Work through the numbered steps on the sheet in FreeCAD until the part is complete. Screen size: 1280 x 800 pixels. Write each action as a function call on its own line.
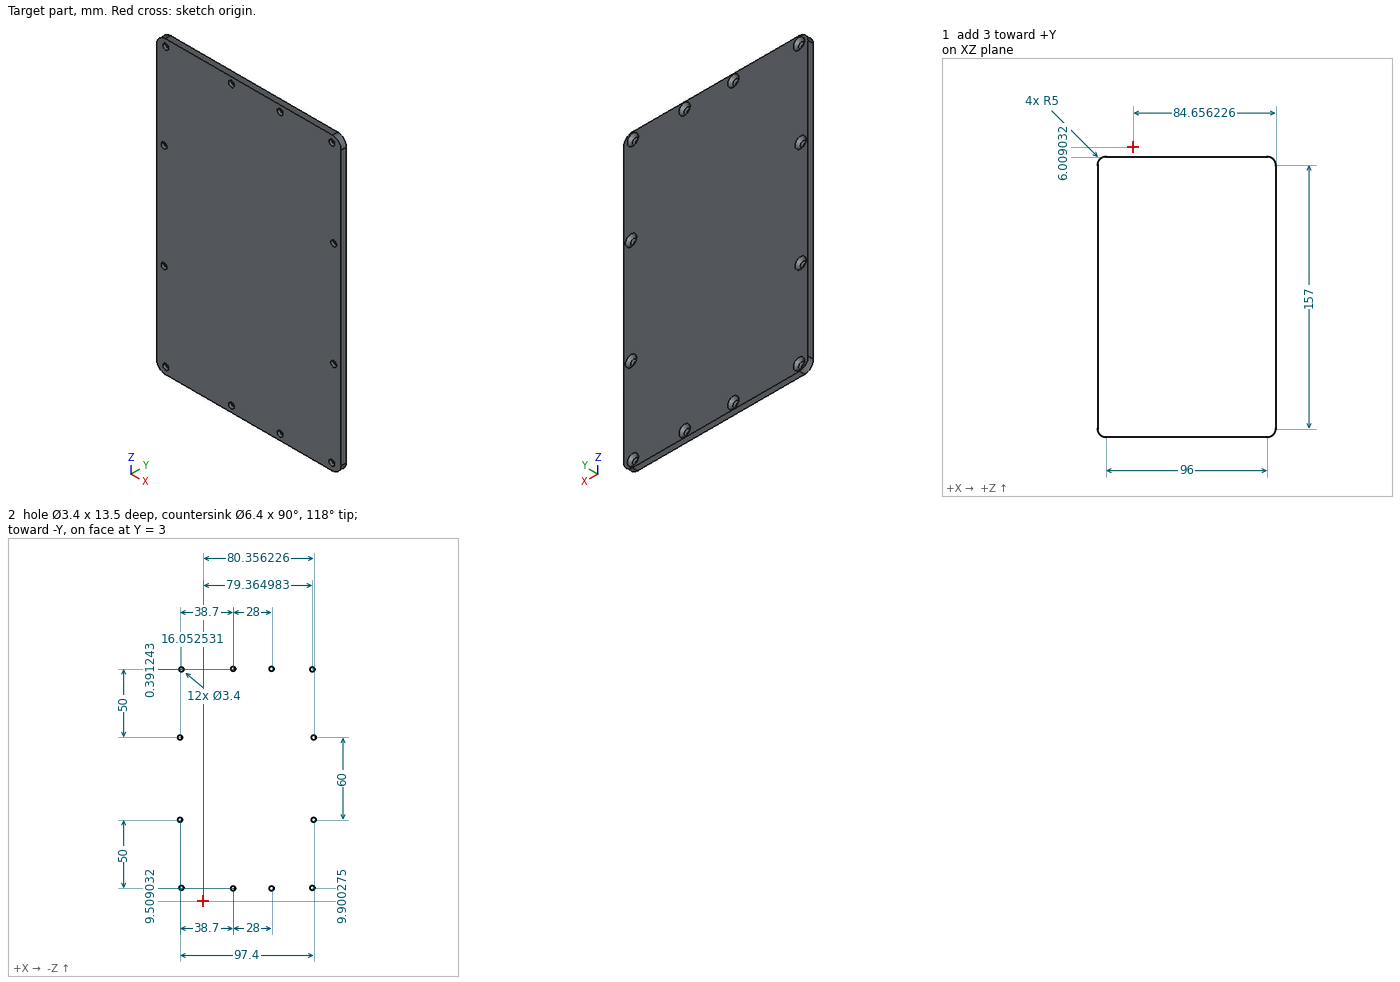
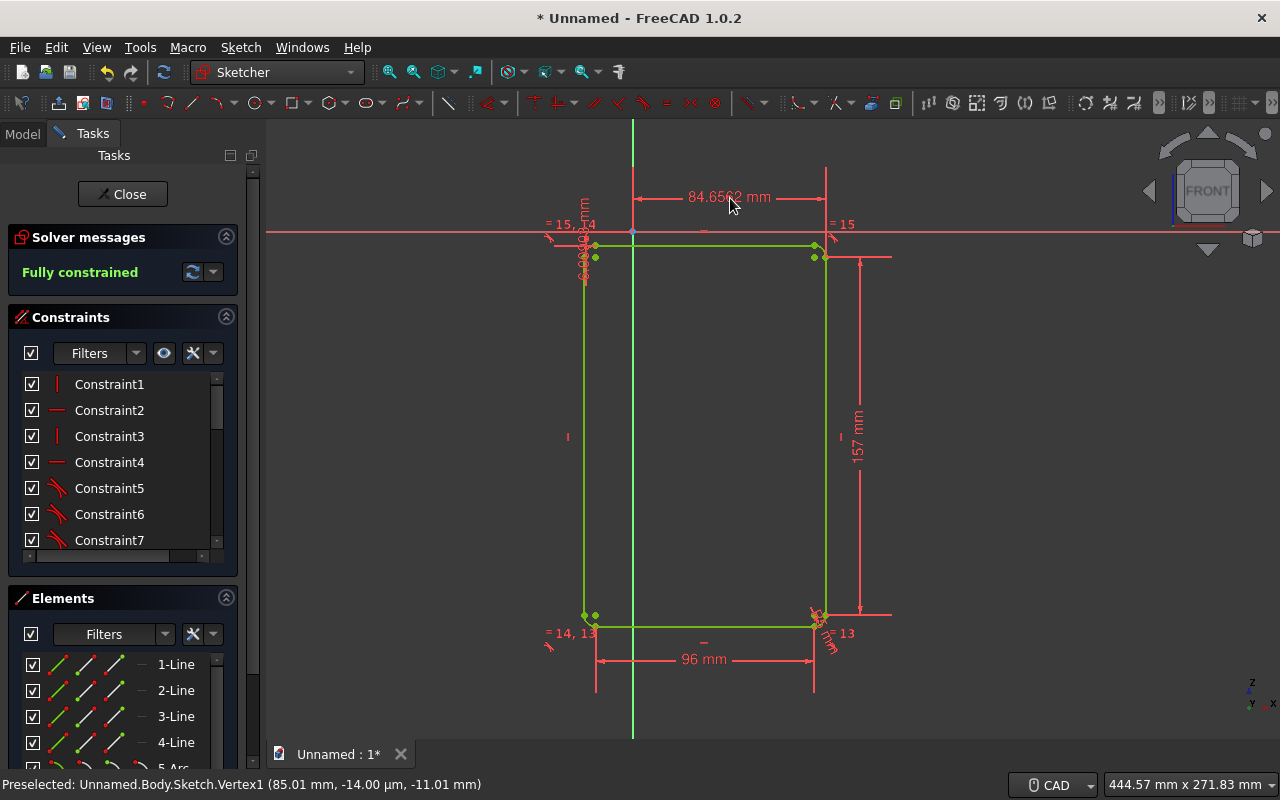
click(123, 194)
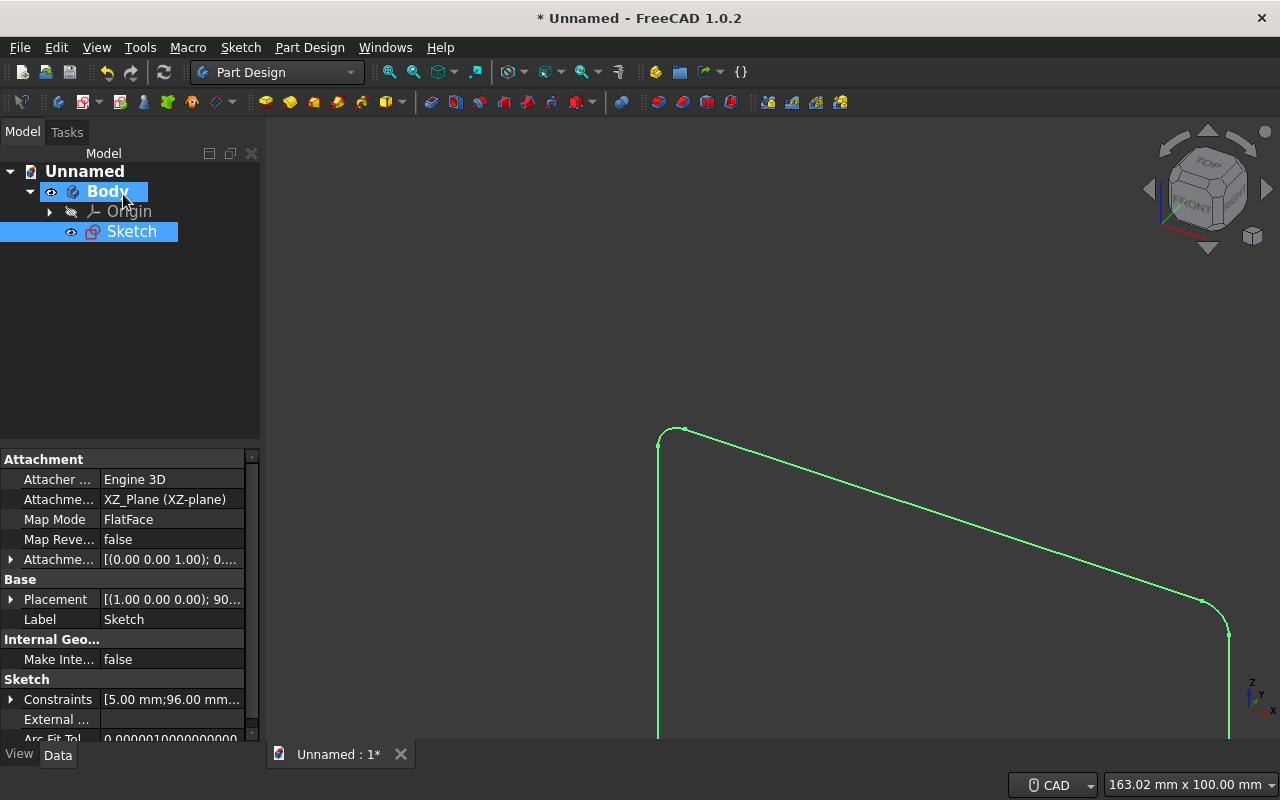
click(266, 102)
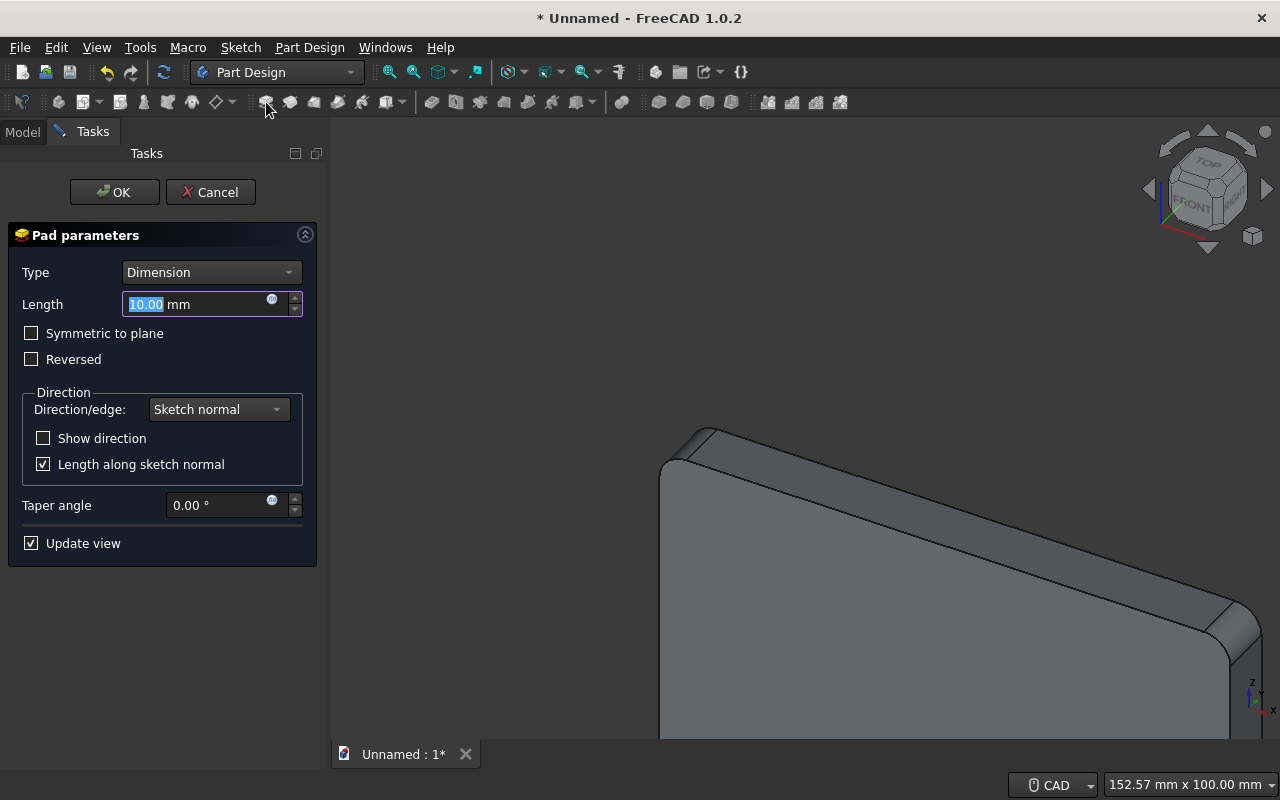
text(3)
key(Tab)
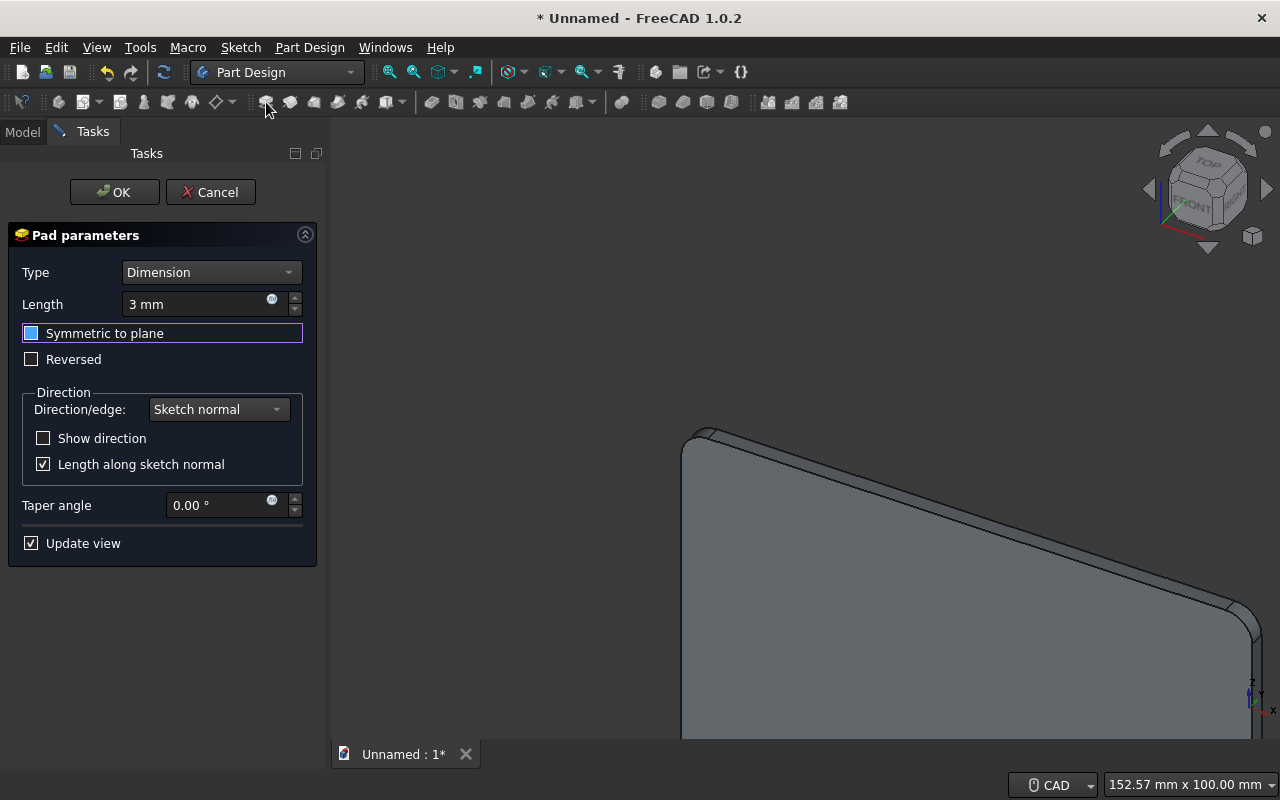
click(30, 359)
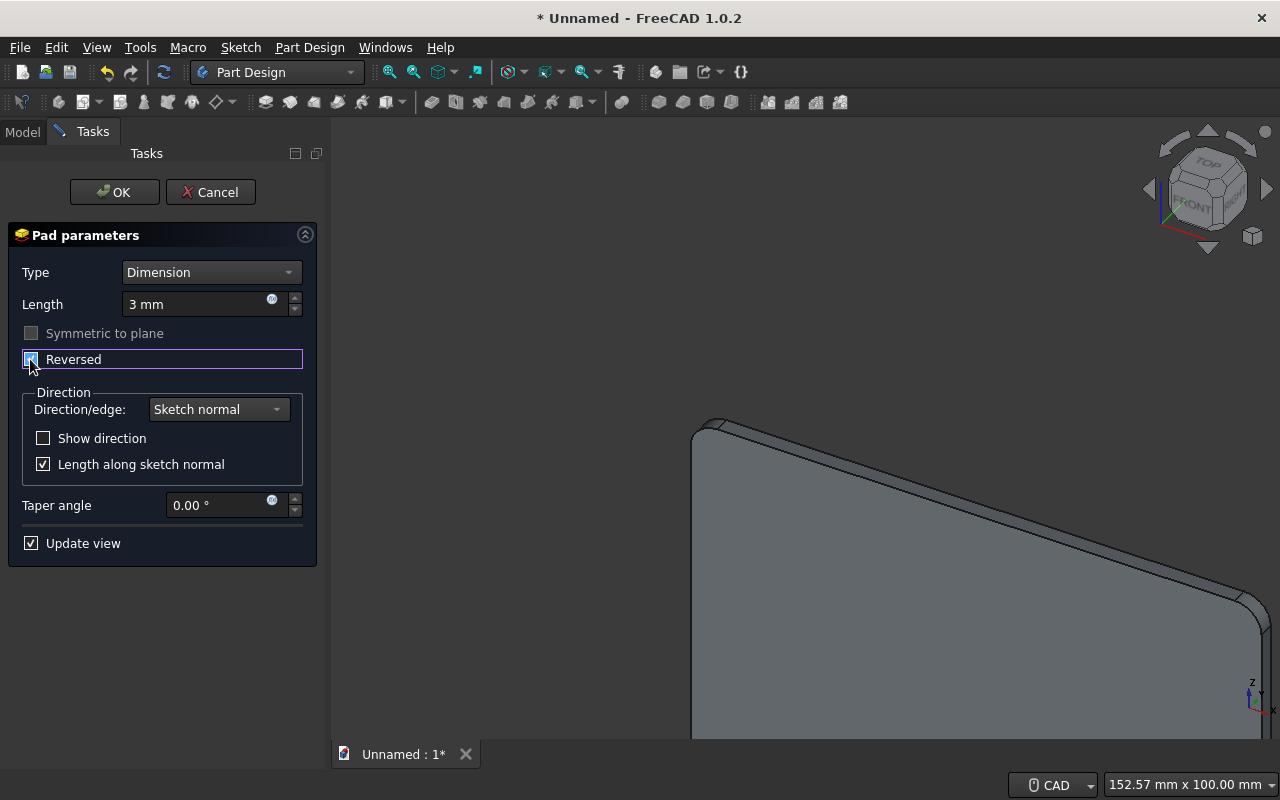
click(115, 192)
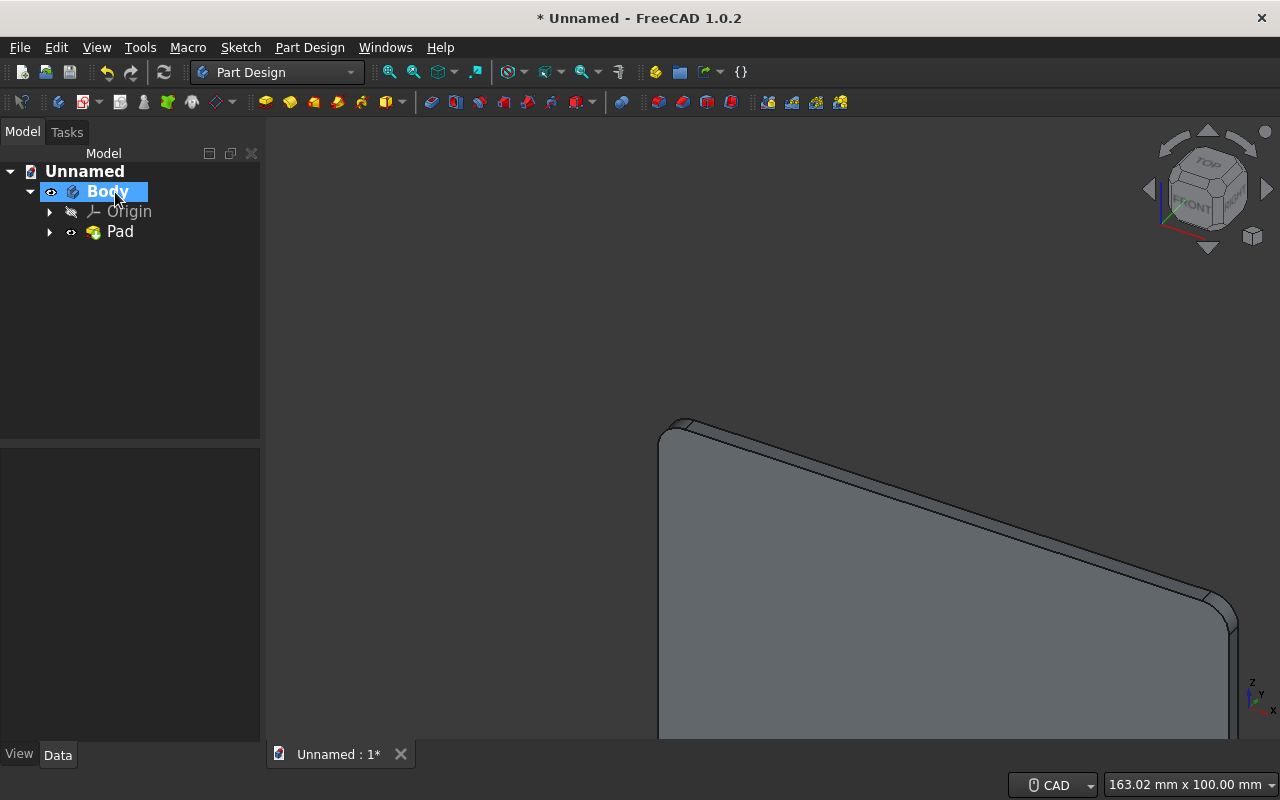
click(390, 72)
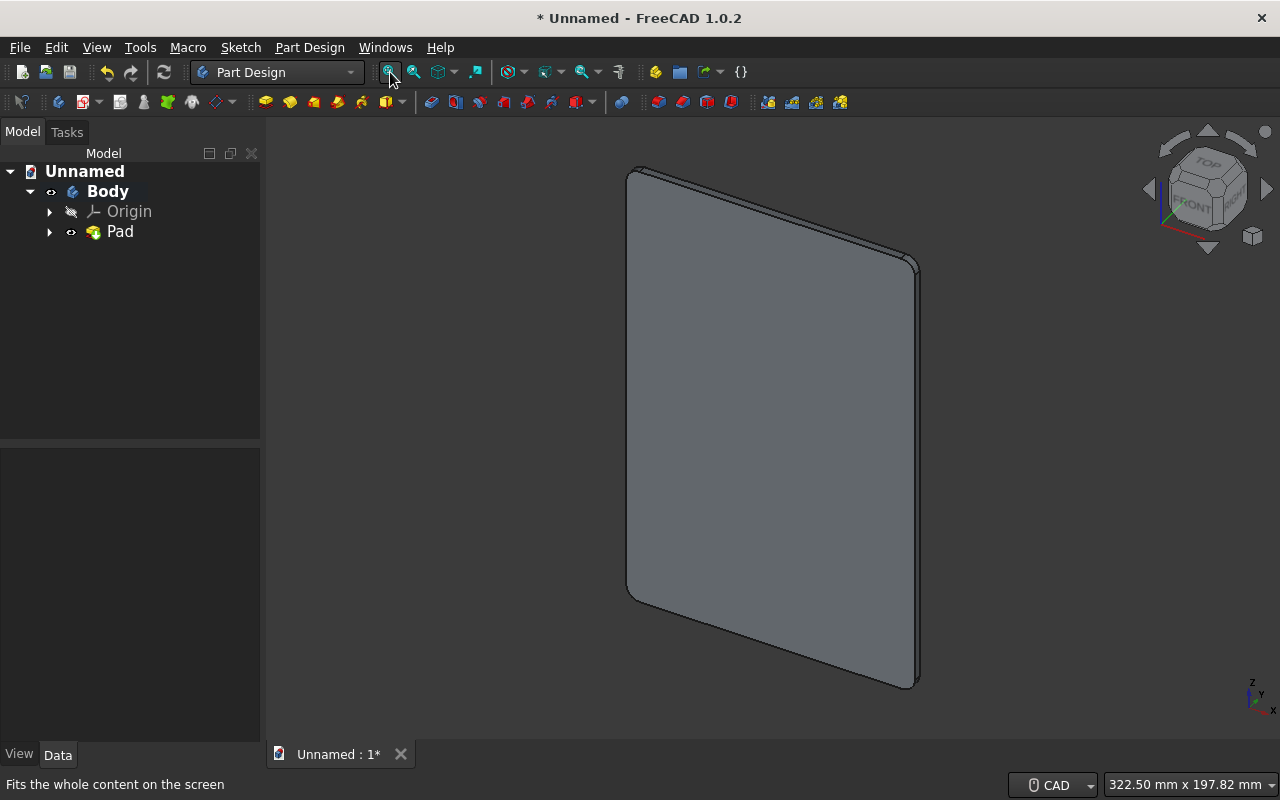
key(4)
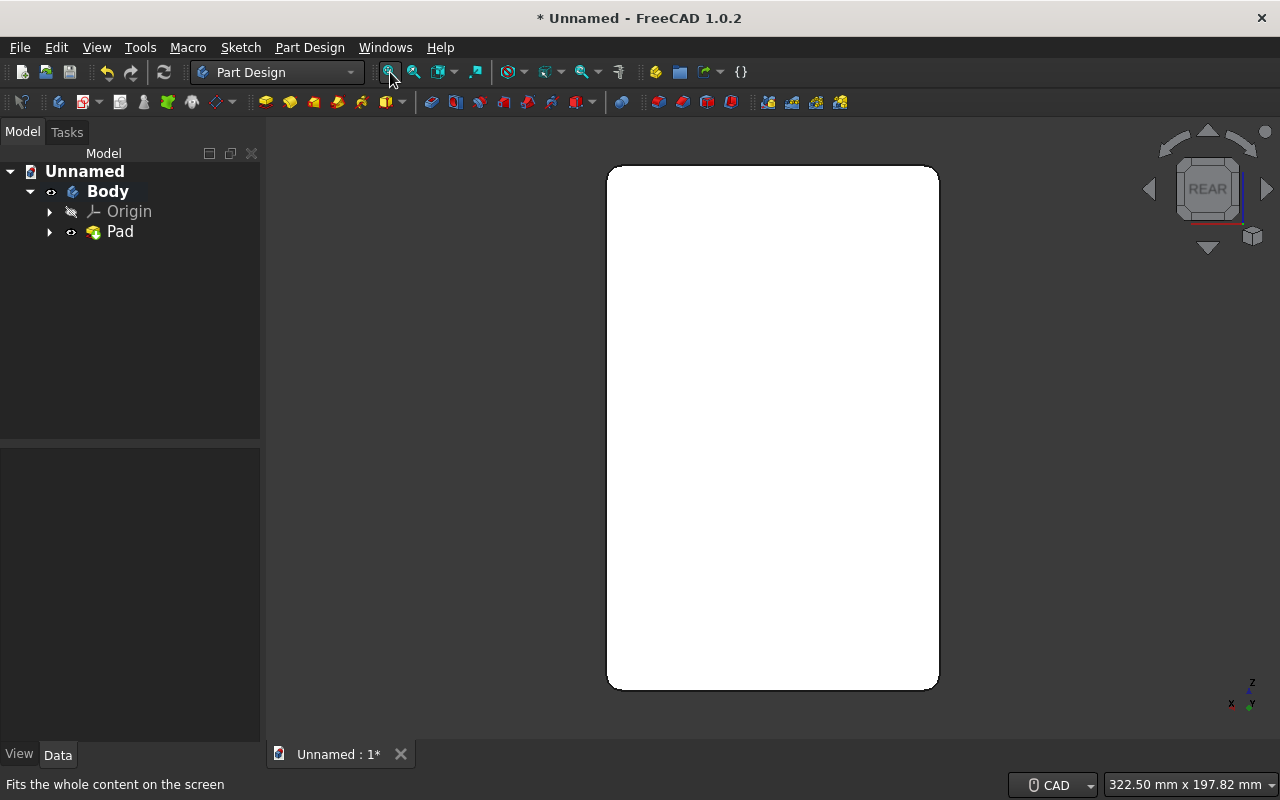
click(773, 352)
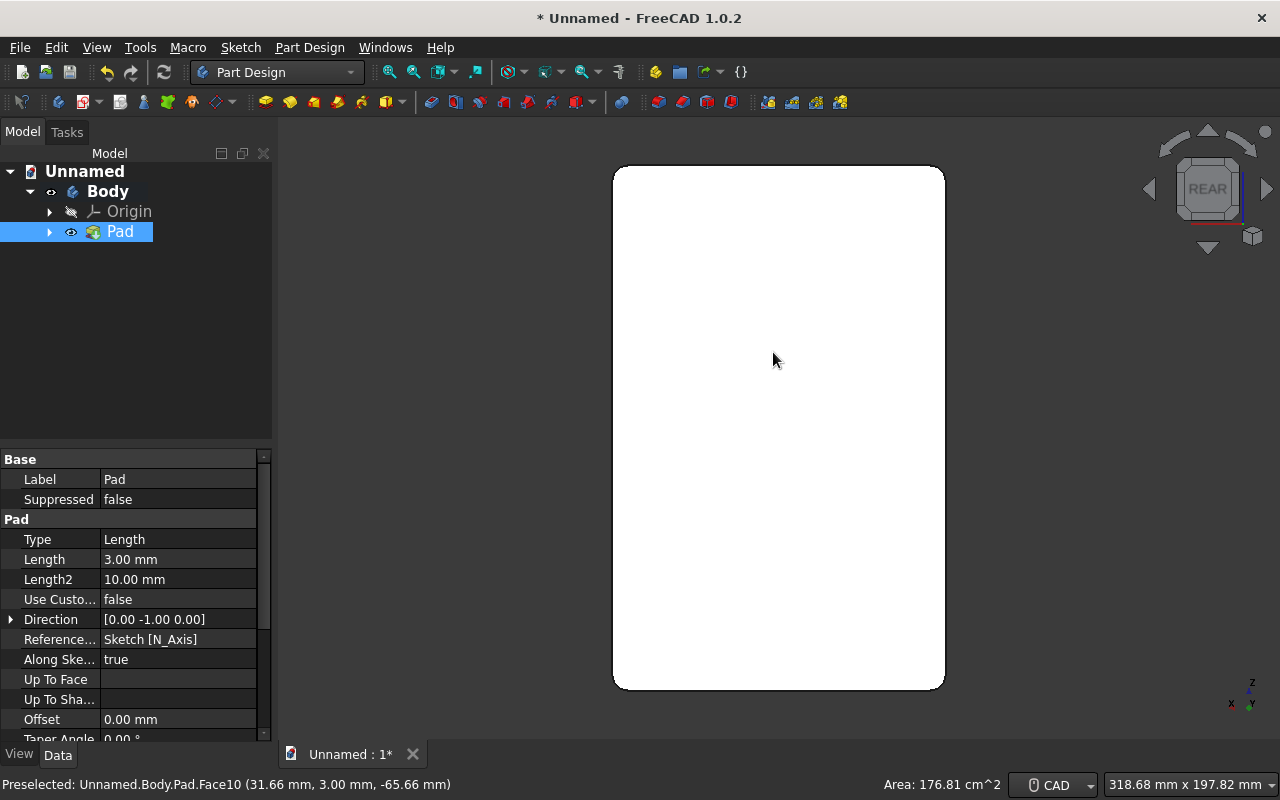
click(84, 102)